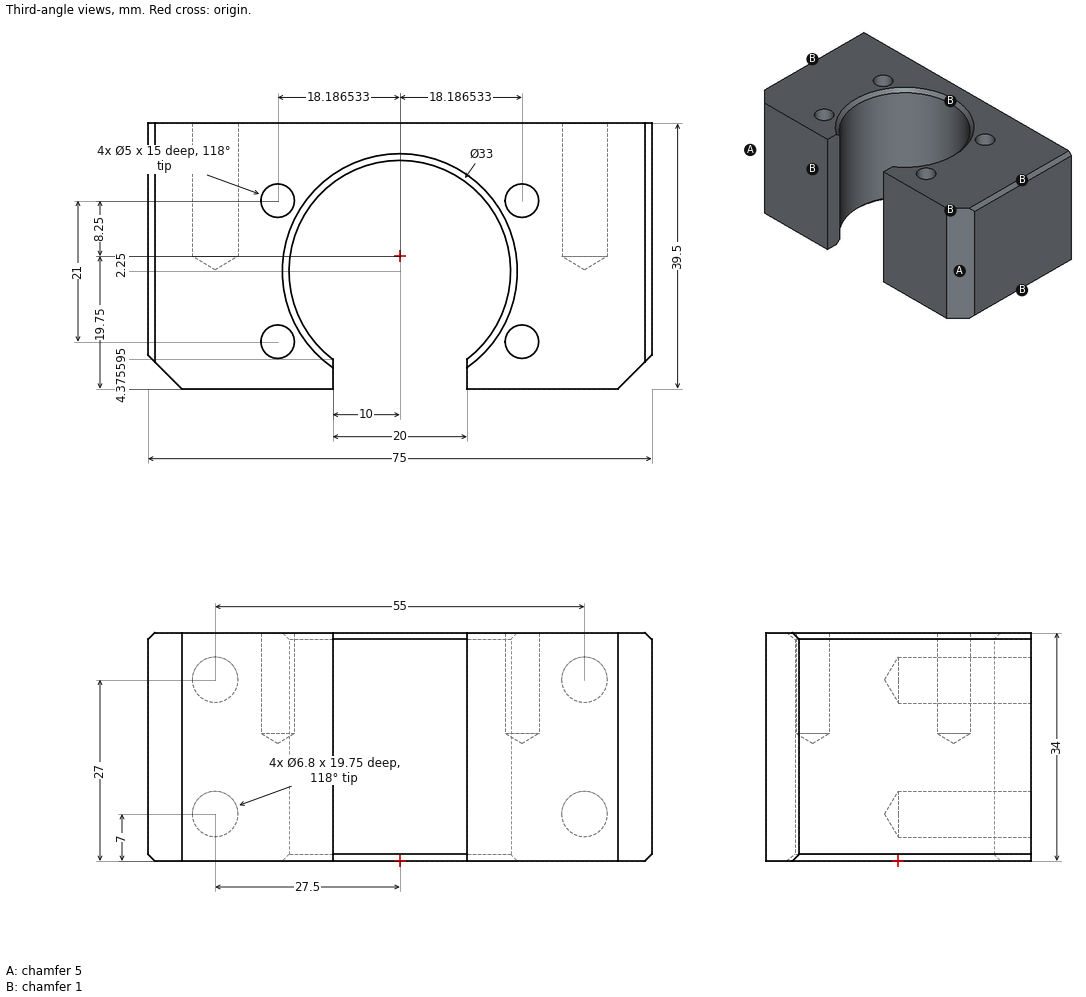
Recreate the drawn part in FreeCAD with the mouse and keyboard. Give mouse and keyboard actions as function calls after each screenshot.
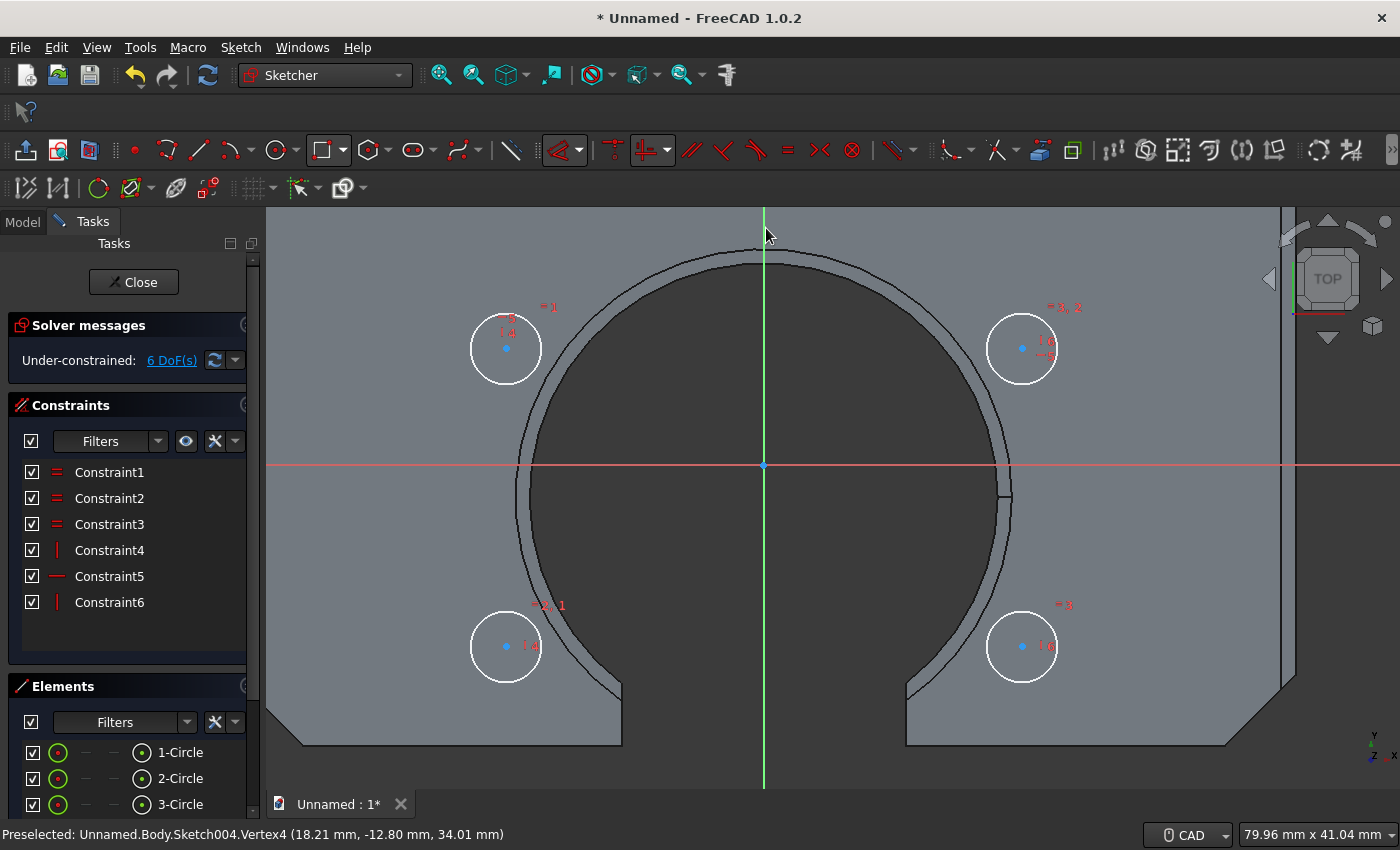
click(506, 647)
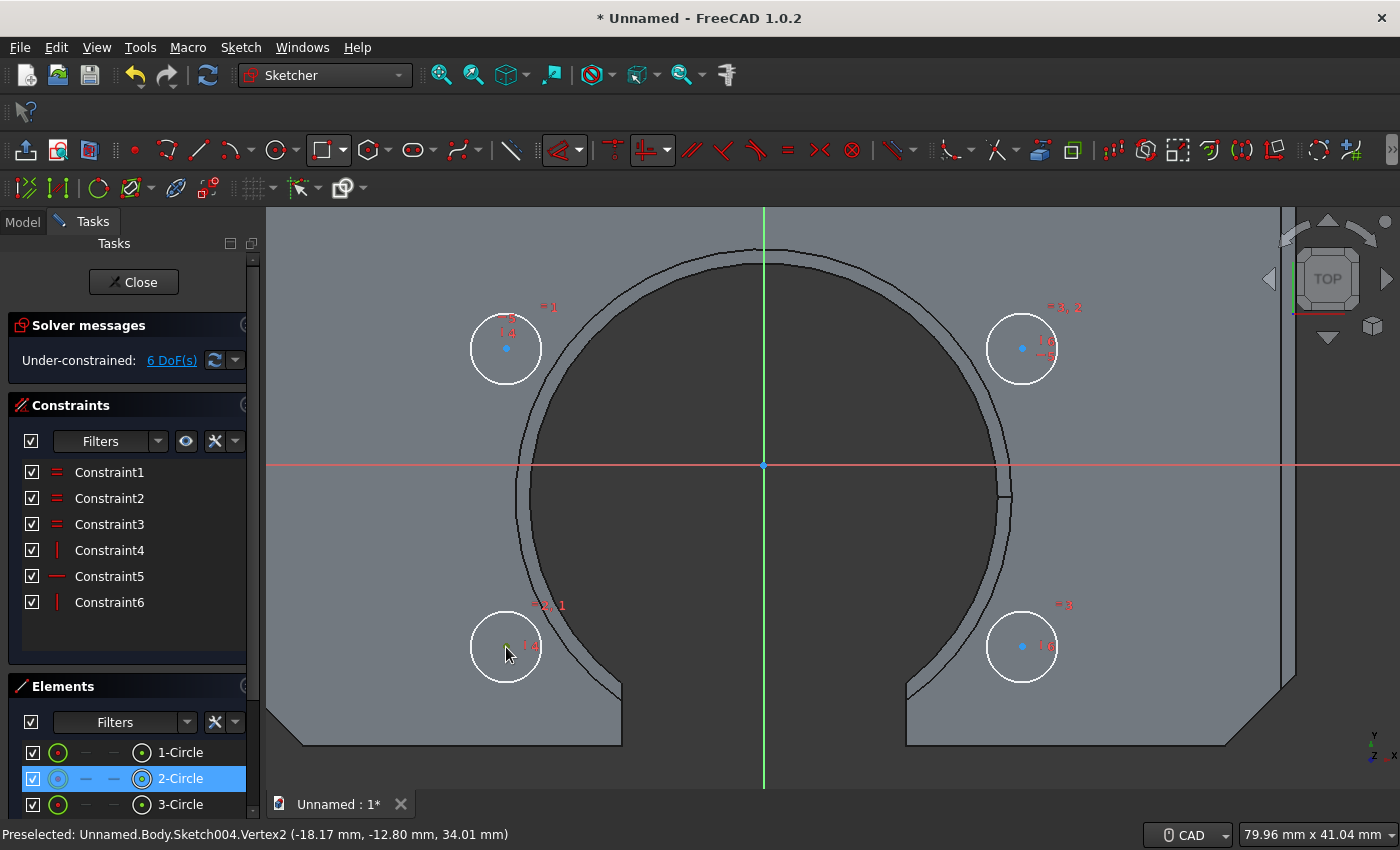
click(1022, 647)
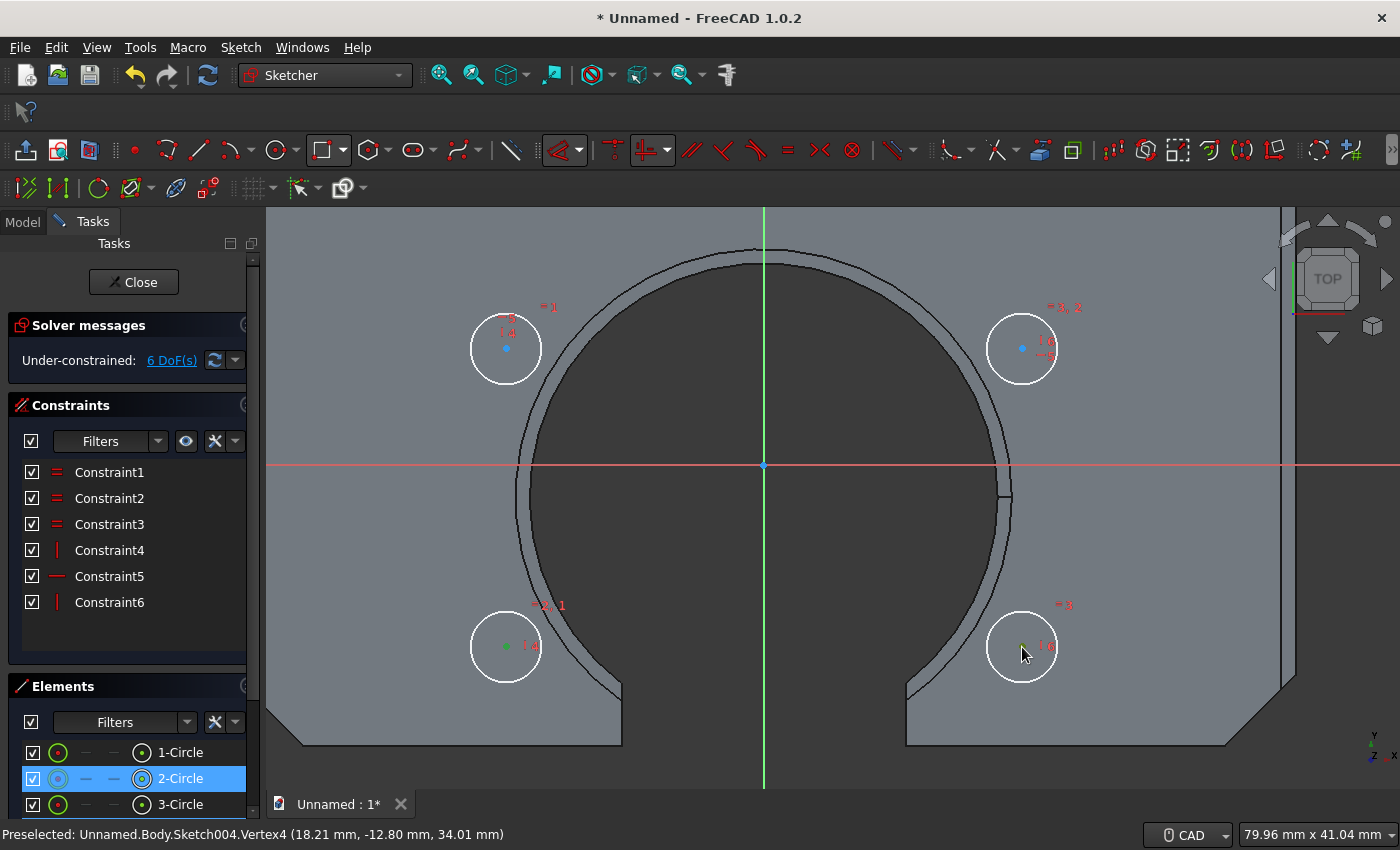
key(h)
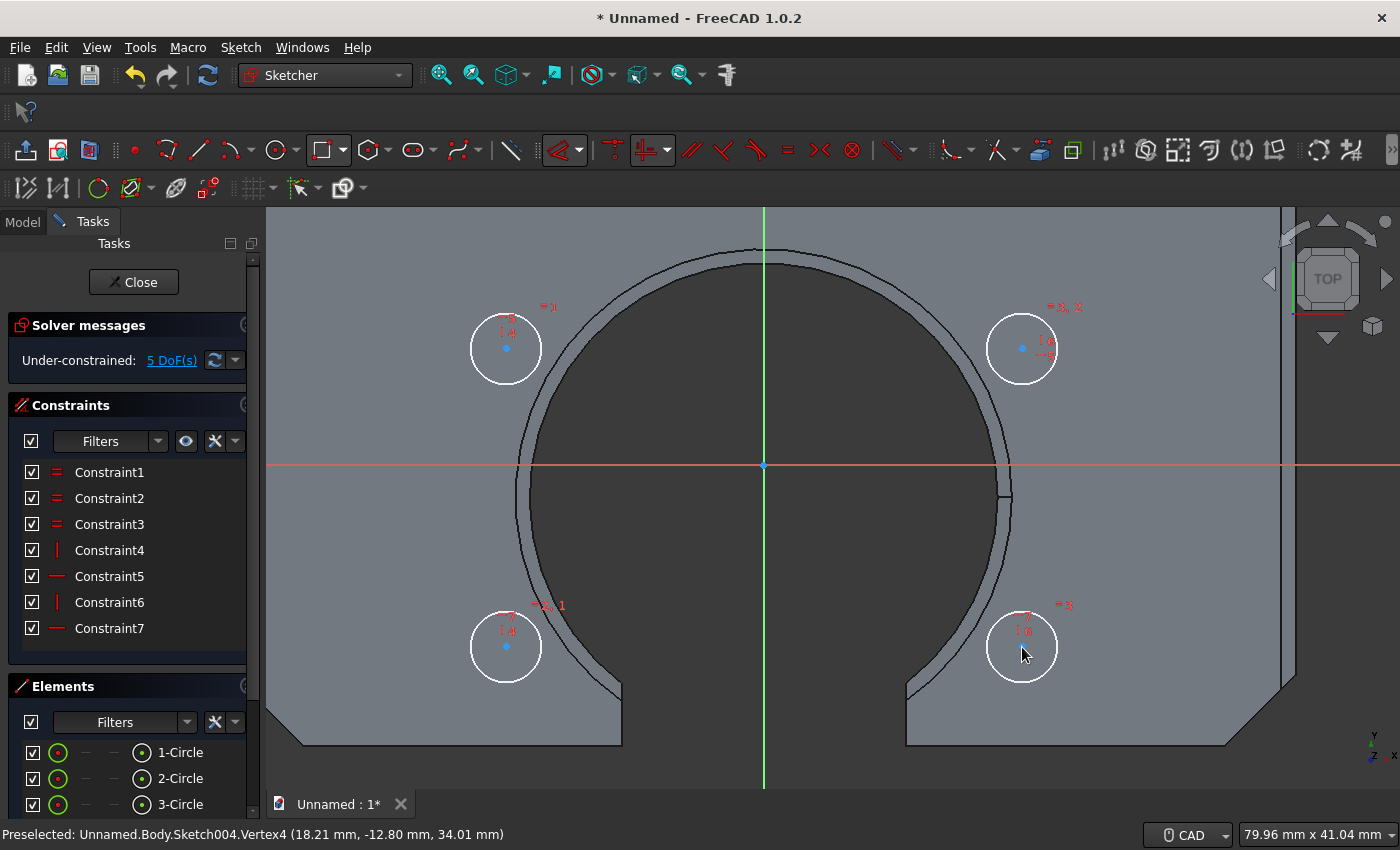
click(531, 324)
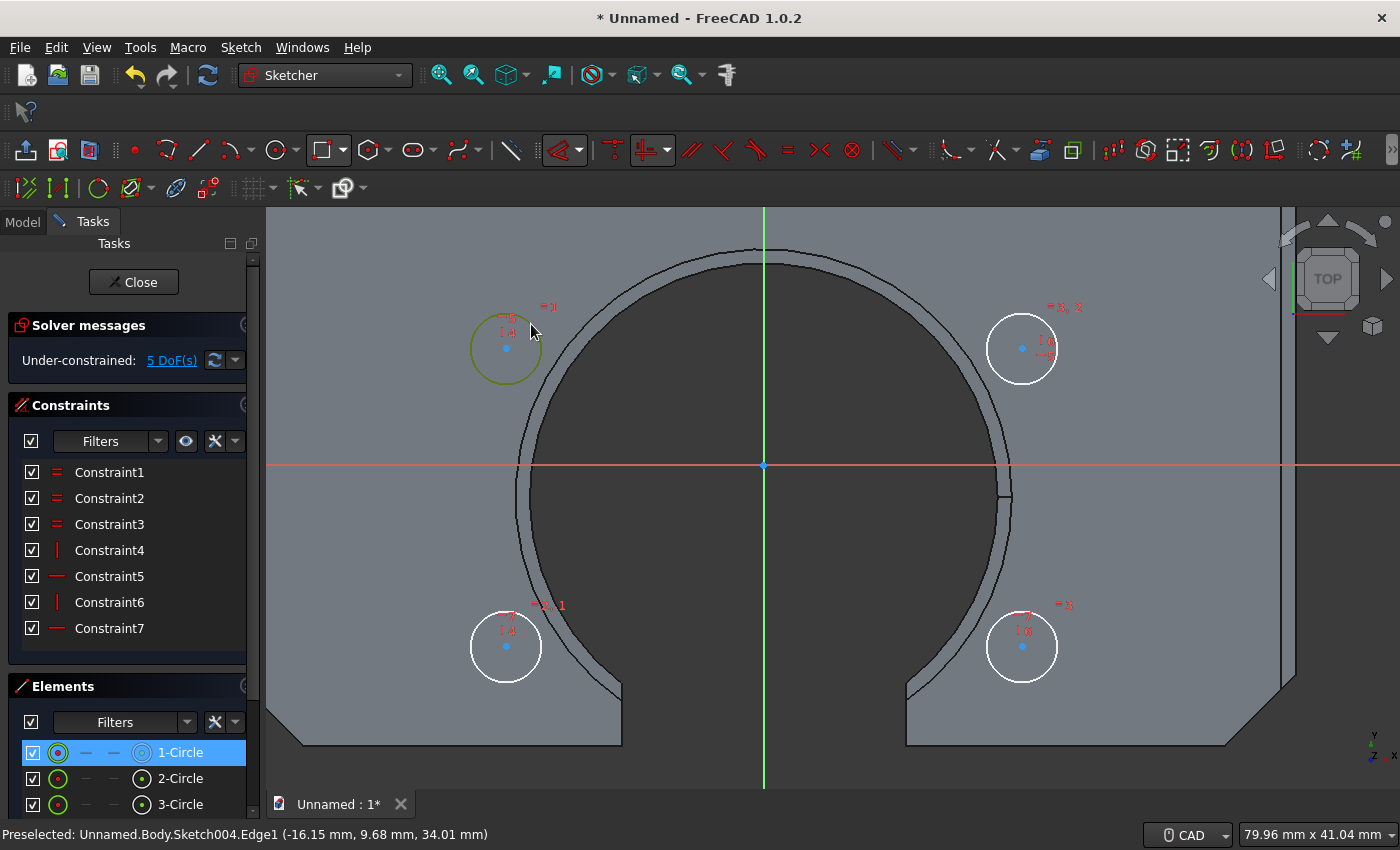
key(k)
key(o)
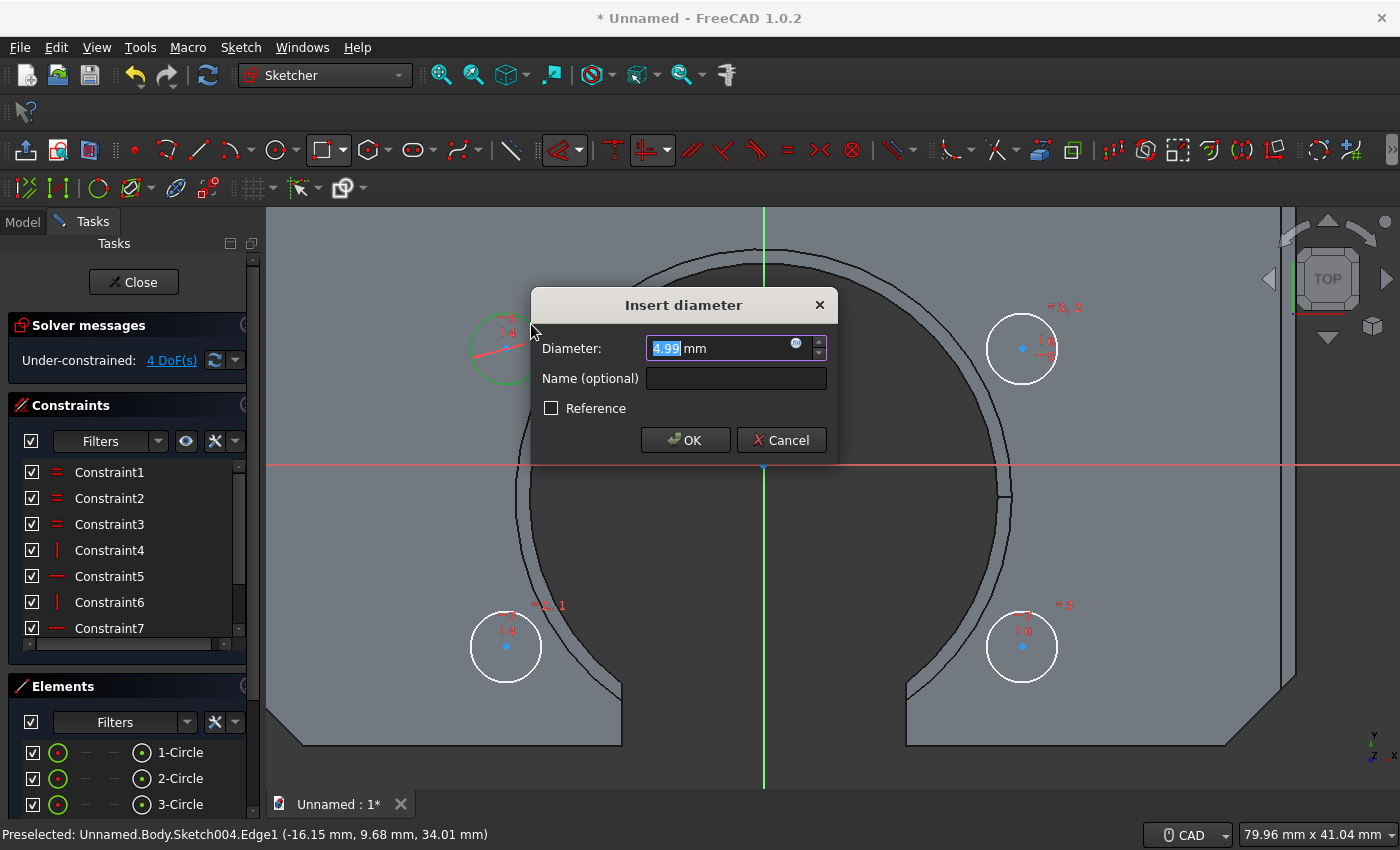
text(5)
key(Return)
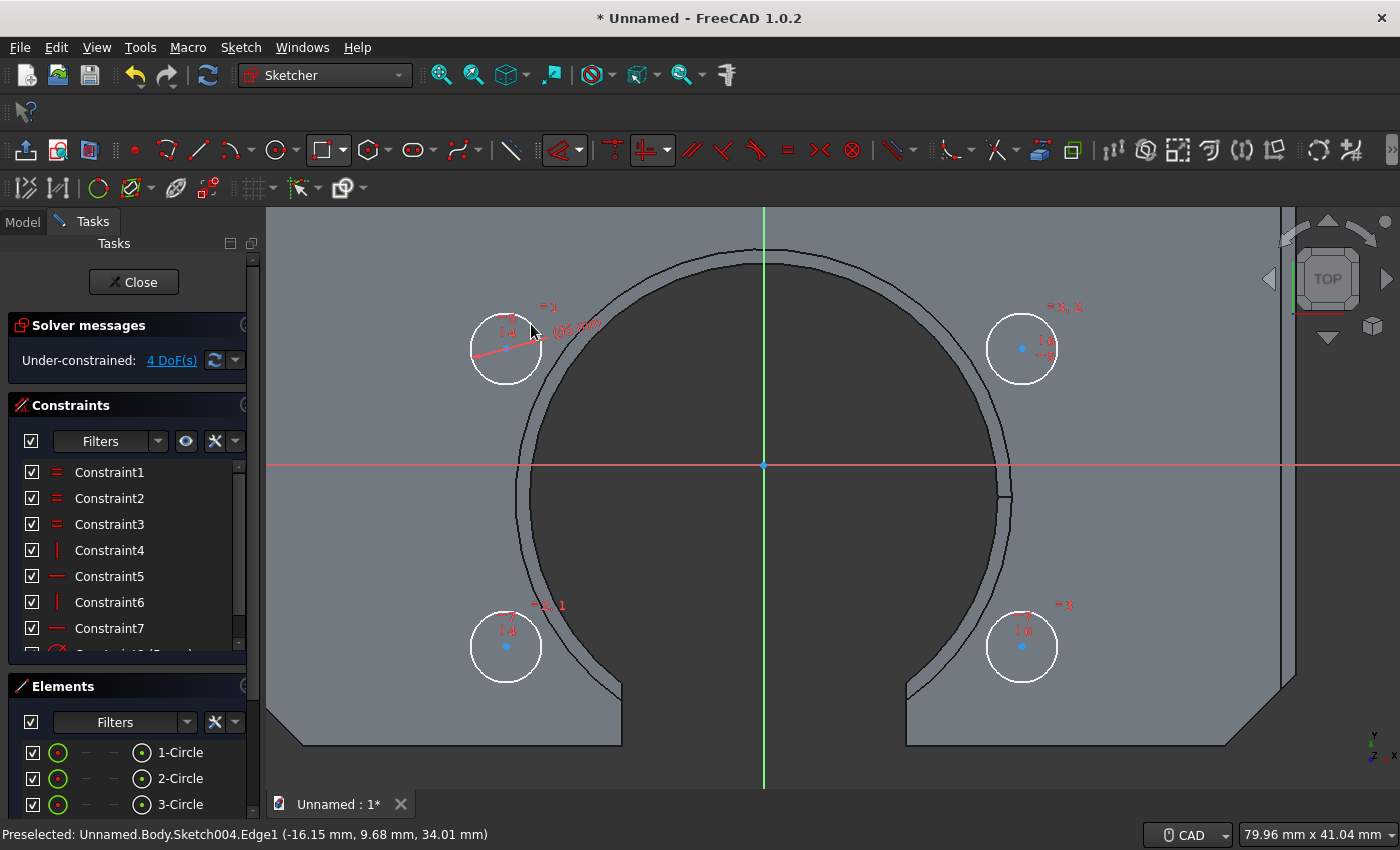
click(506, 349)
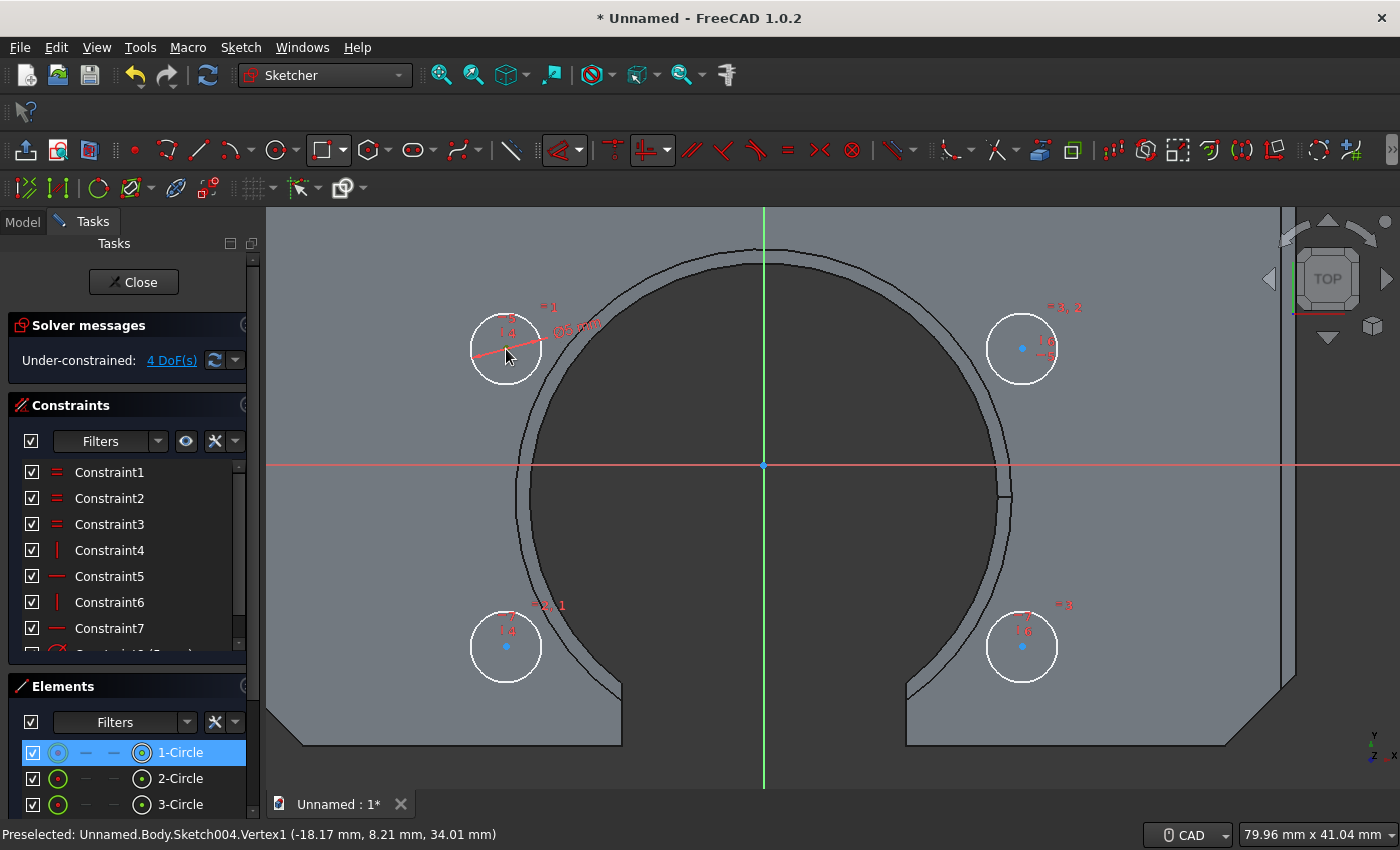
click(506, 647)